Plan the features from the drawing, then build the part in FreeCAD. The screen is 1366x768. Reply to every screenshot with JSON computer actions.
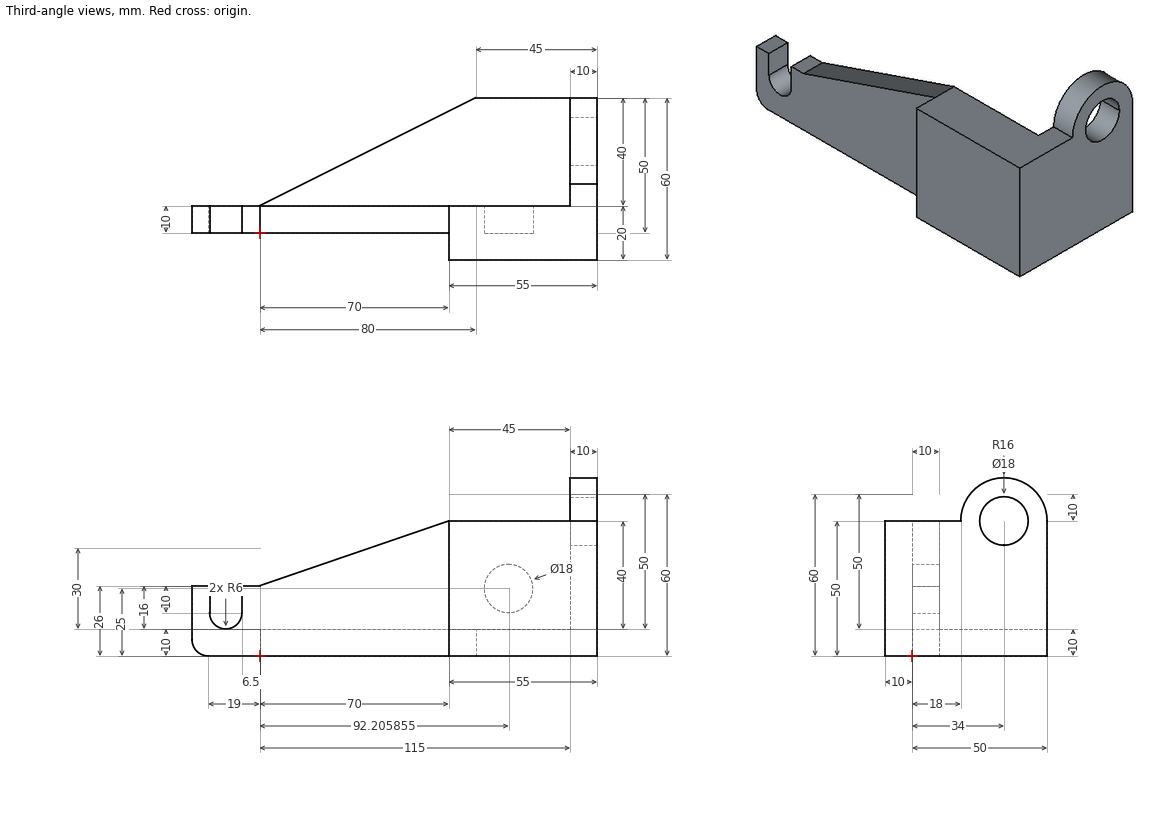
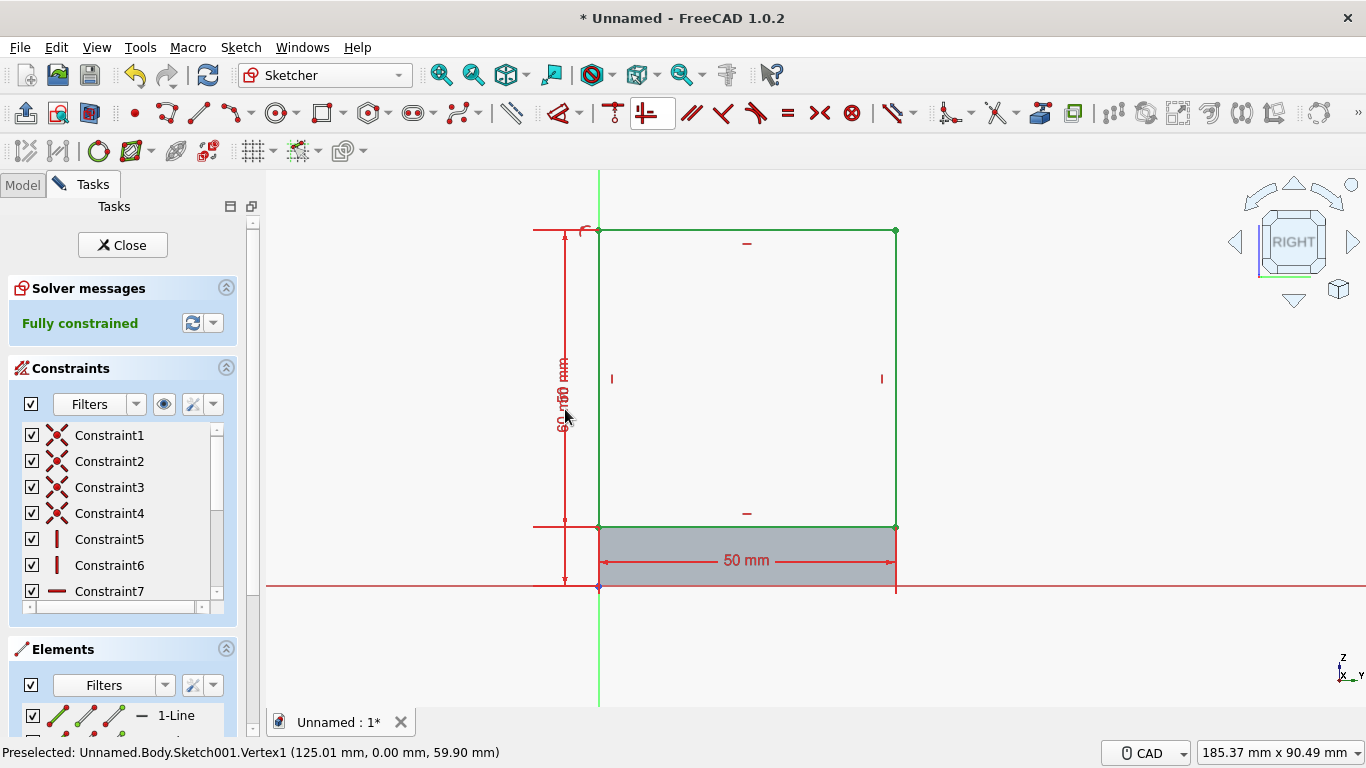
{"action": "left_click", "coordinate": [123, 245]}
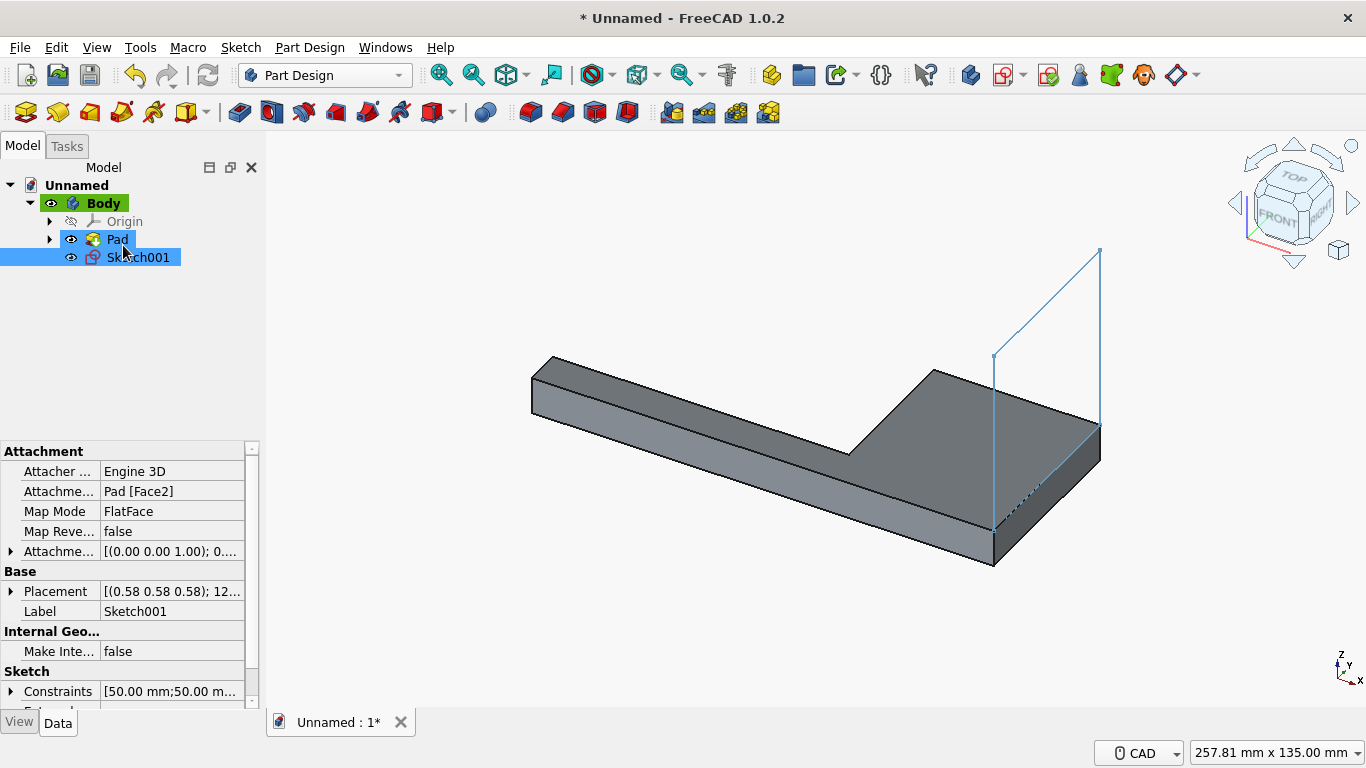
{"action": "left_click", "coordinate": [26, 112]}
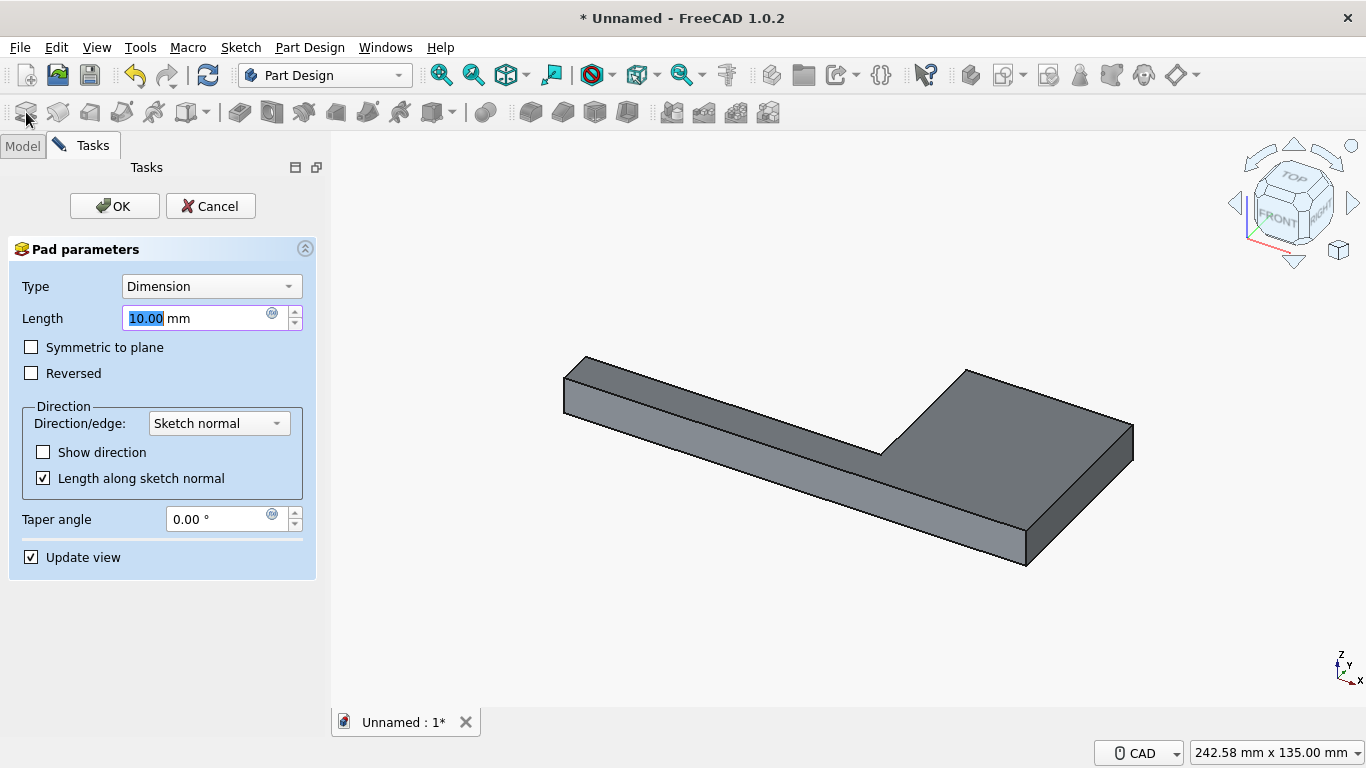
{"action": "type", "text": "10"}
{"action": "key", "text": "Tab"}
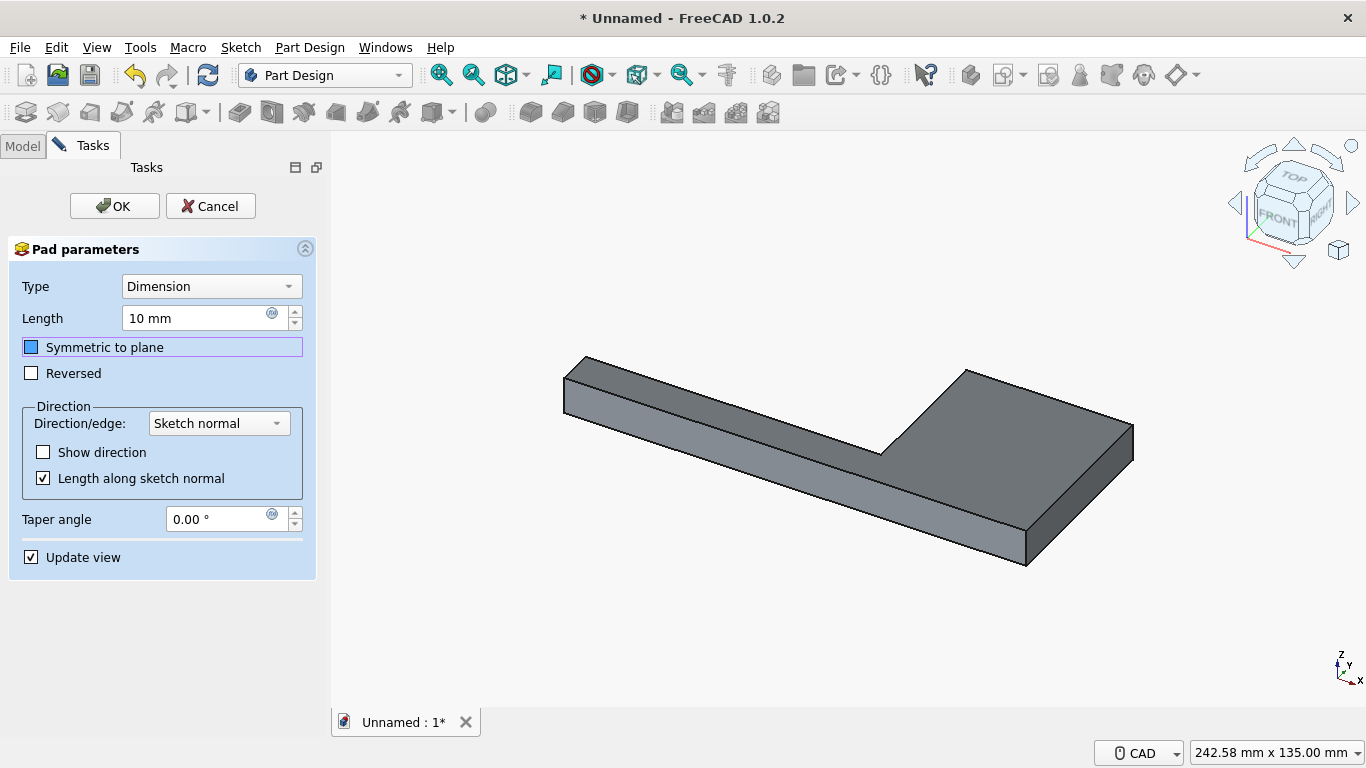
{"action": "left_click", "coordinate": [30, 373]}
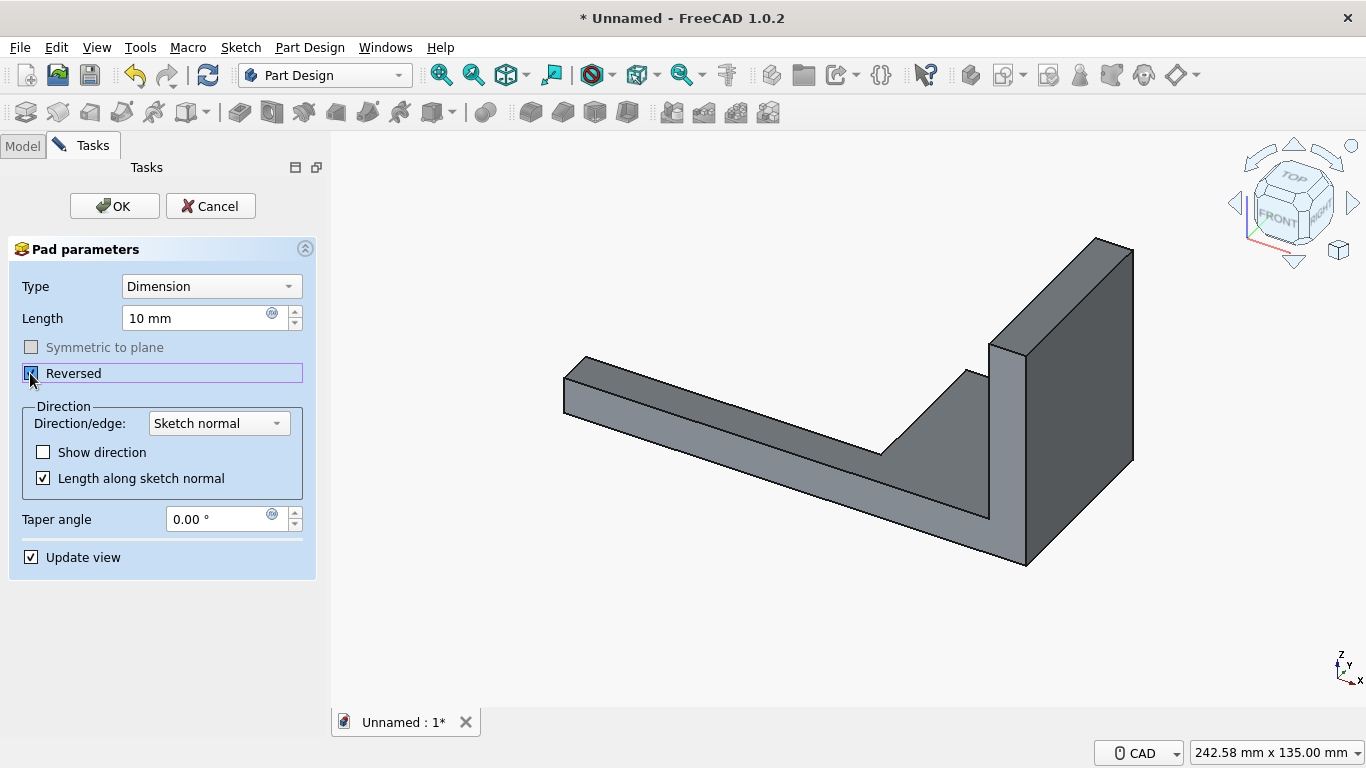
{"action": "left_click", "coordinate": [115, 206]}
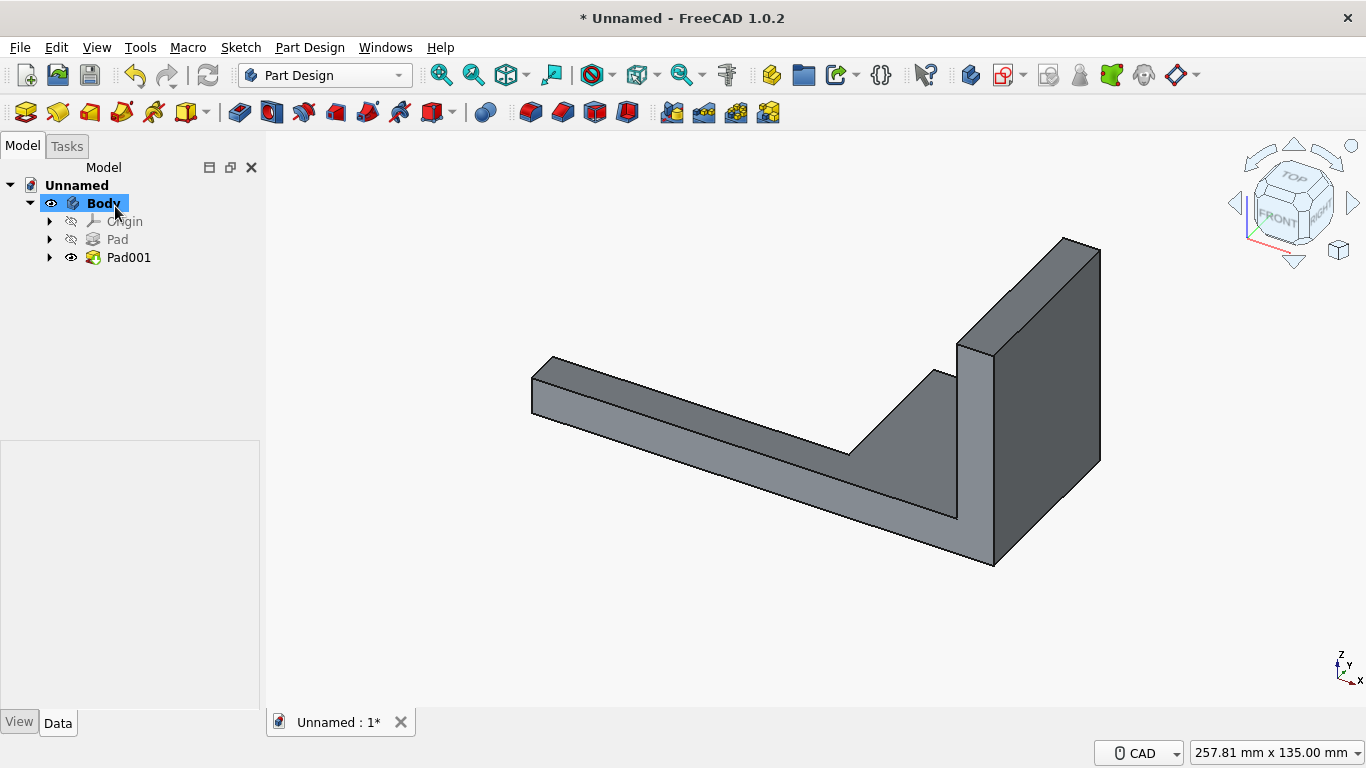
{"action": "left_click", "coordinate": [442, 76]}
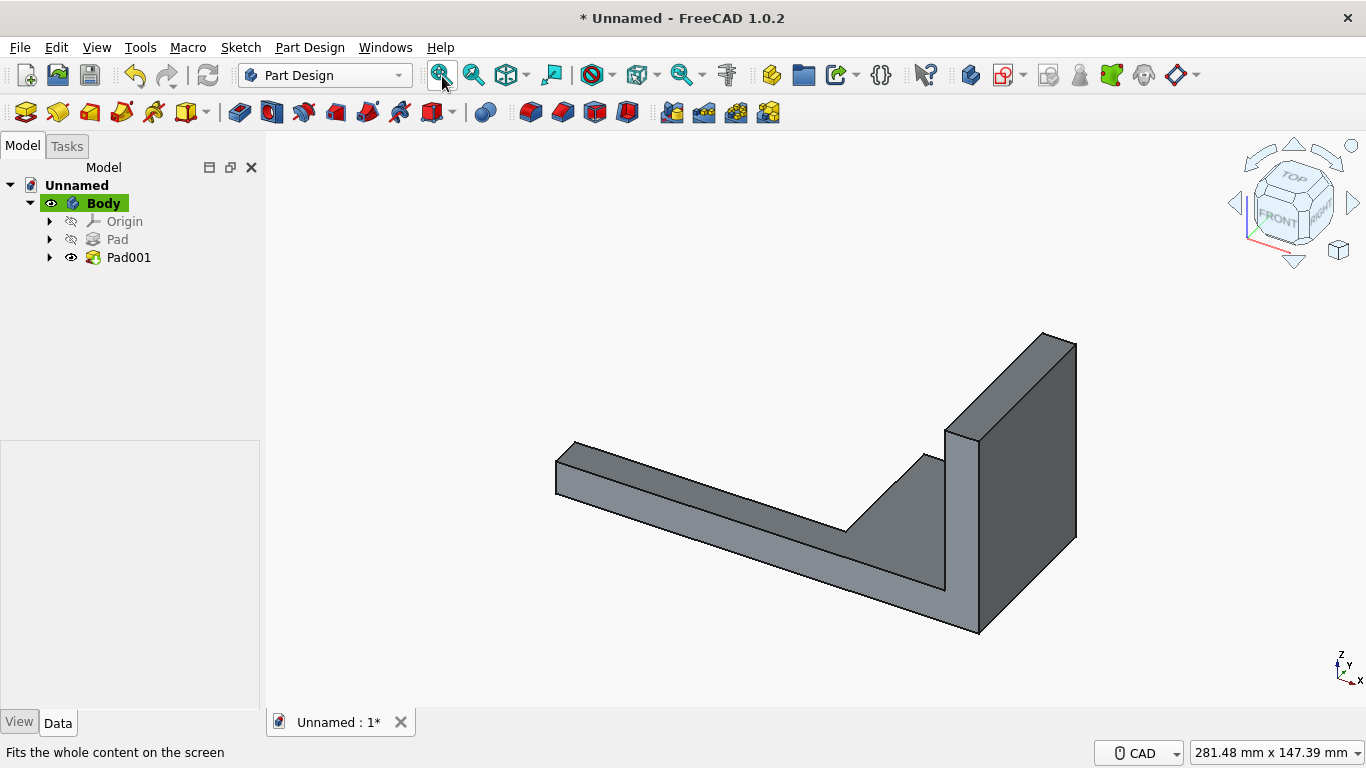
{"action": "left_click", "coordinate": [948, 609]}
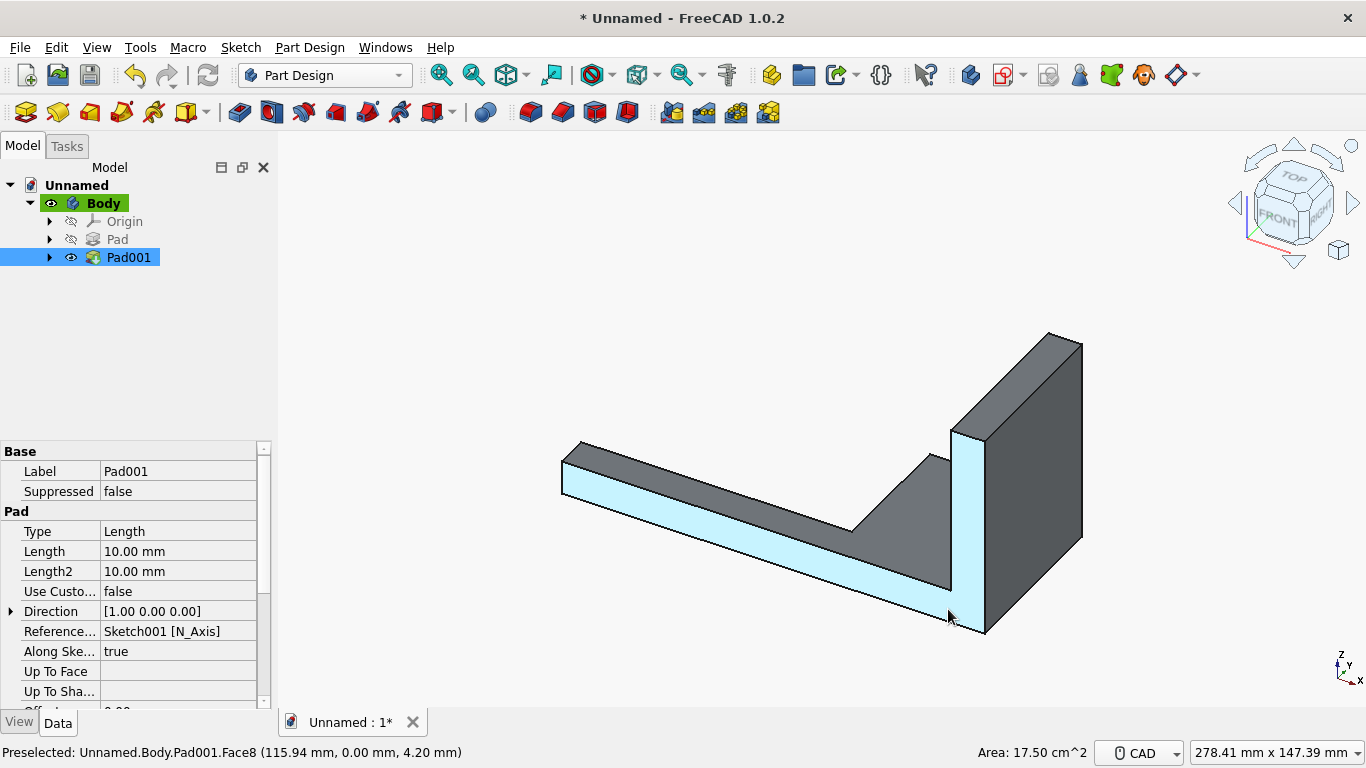
{"action": "left_click", "coordinate": [1004, 76]}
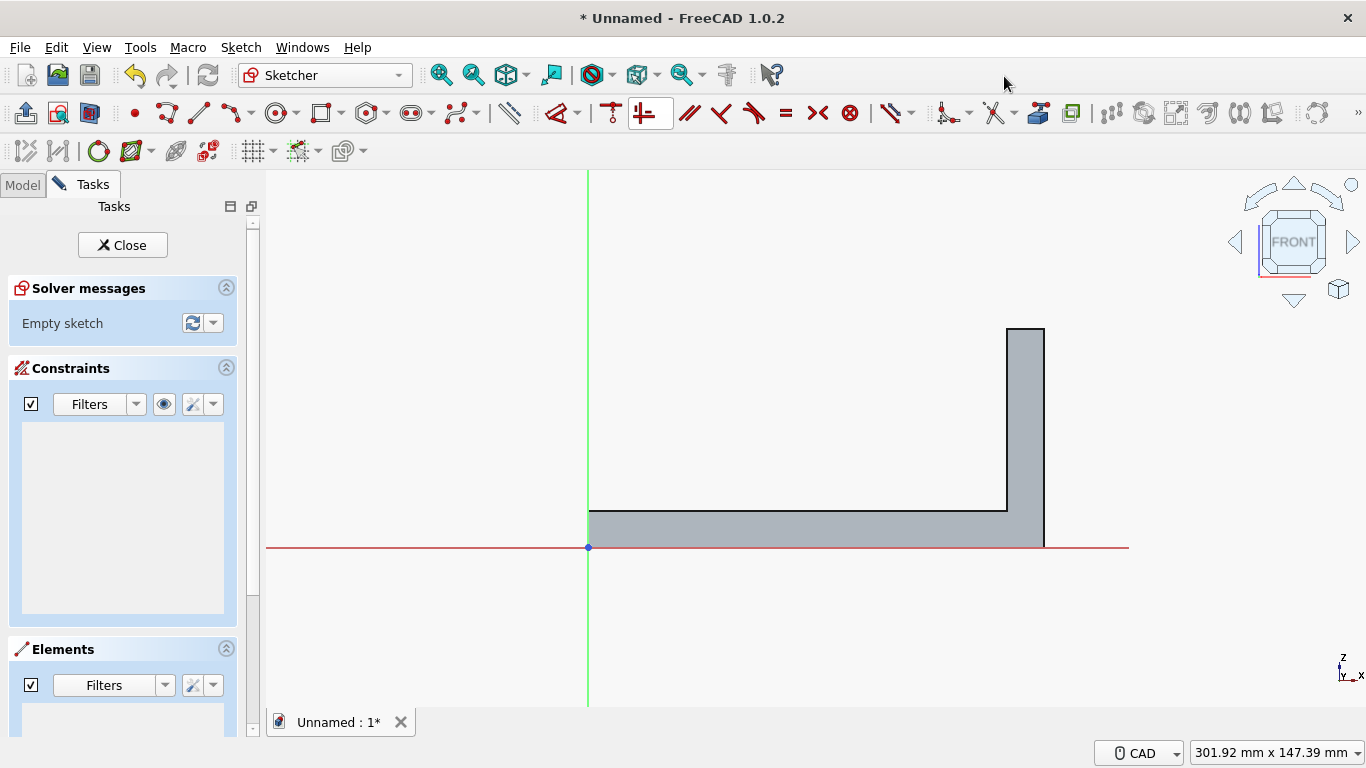
{"action": "scroll", "coordinate": [900, 439], "scroll_direction": "up", "scroll_amount": 2}